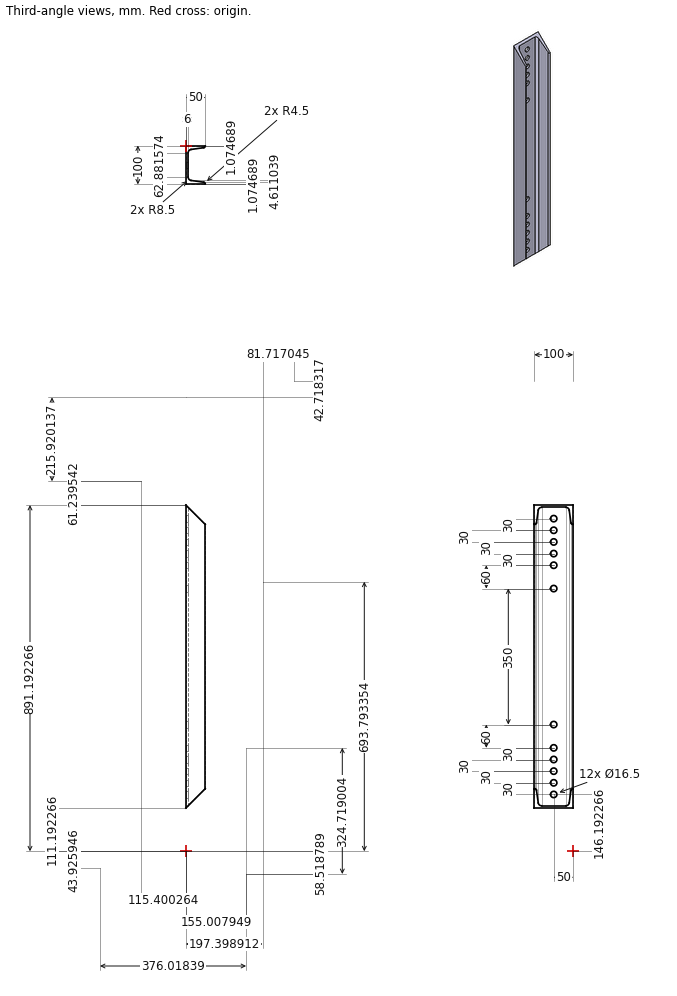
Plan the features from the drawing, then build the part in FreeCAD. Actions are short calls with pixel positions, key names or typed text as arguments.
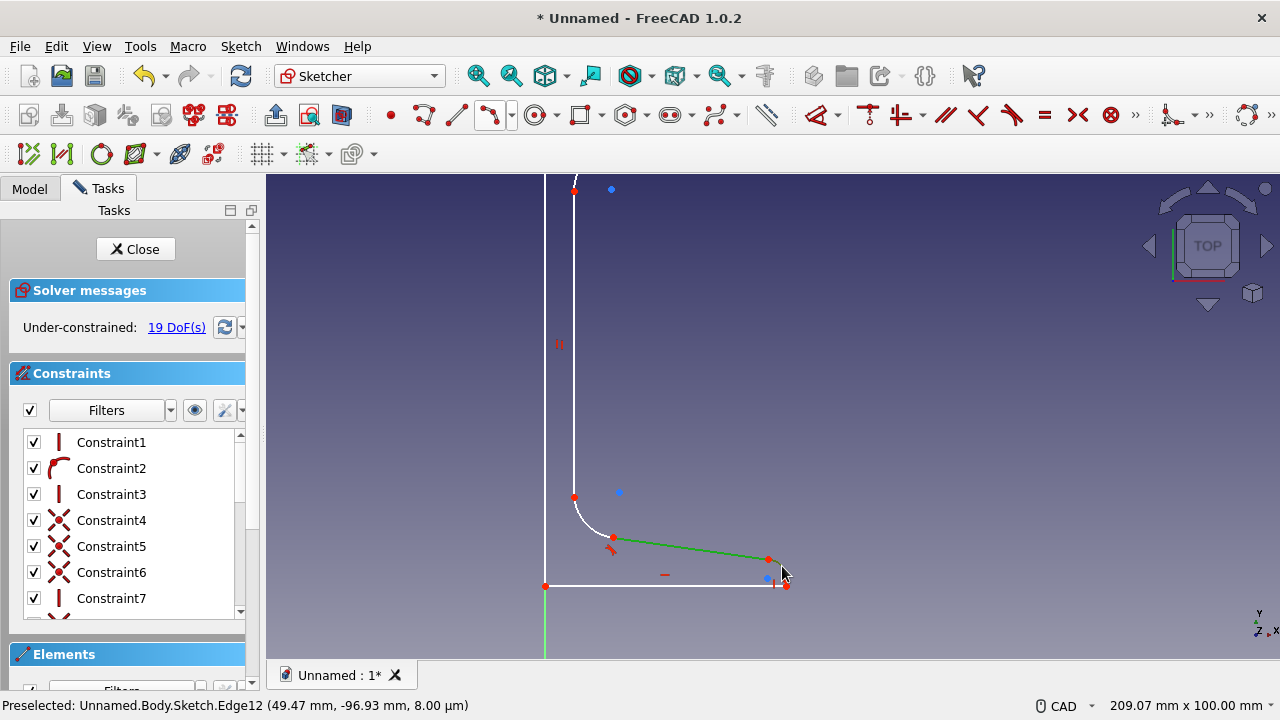
click(1012, 116)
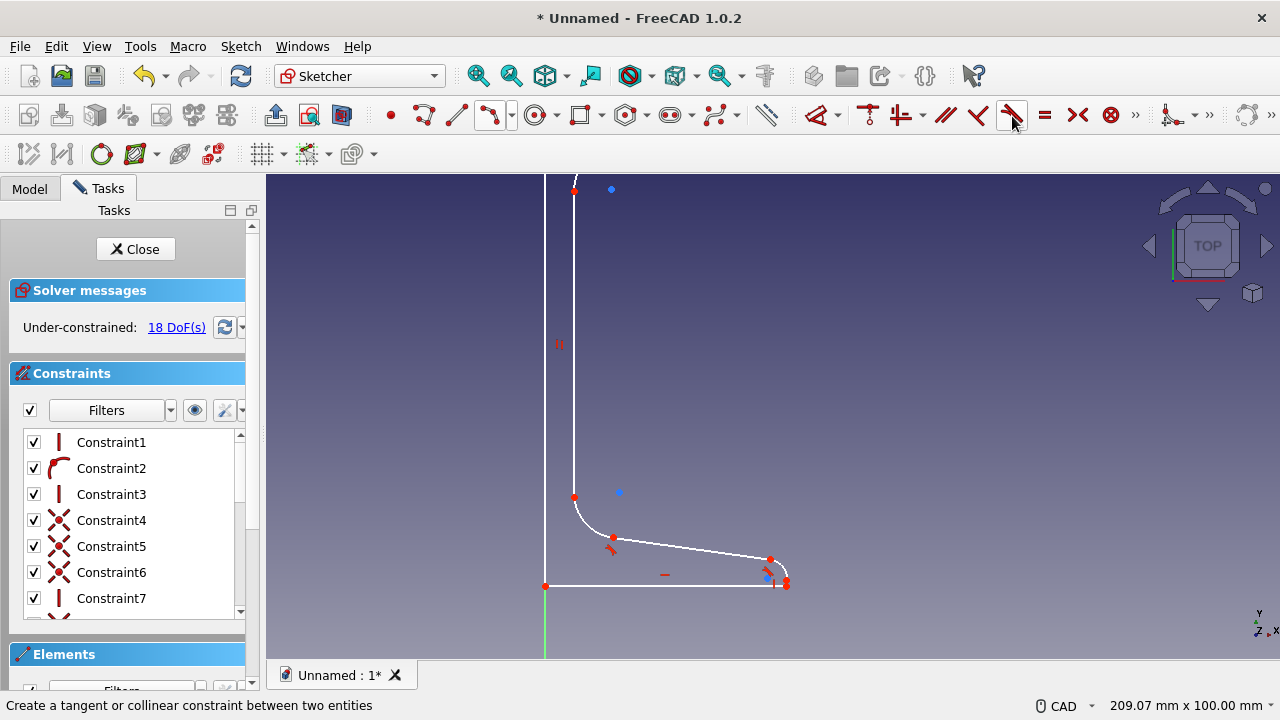
click(574, 406)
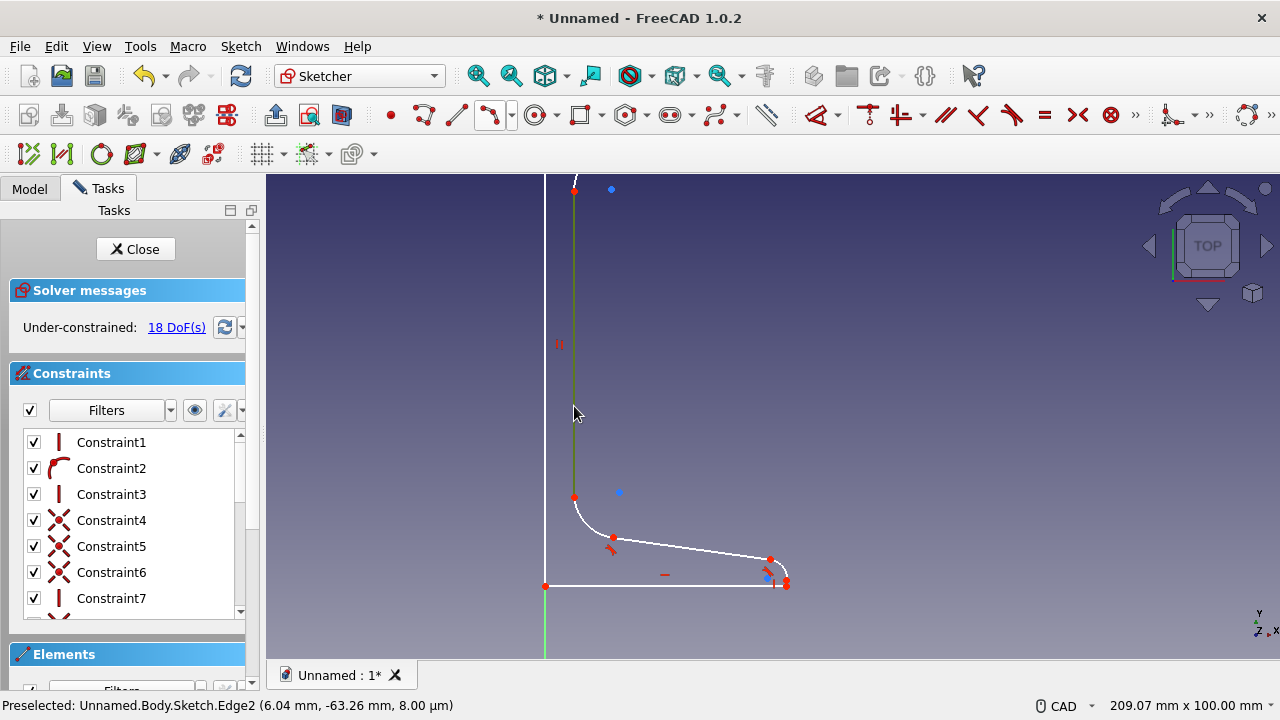
click(580, 515)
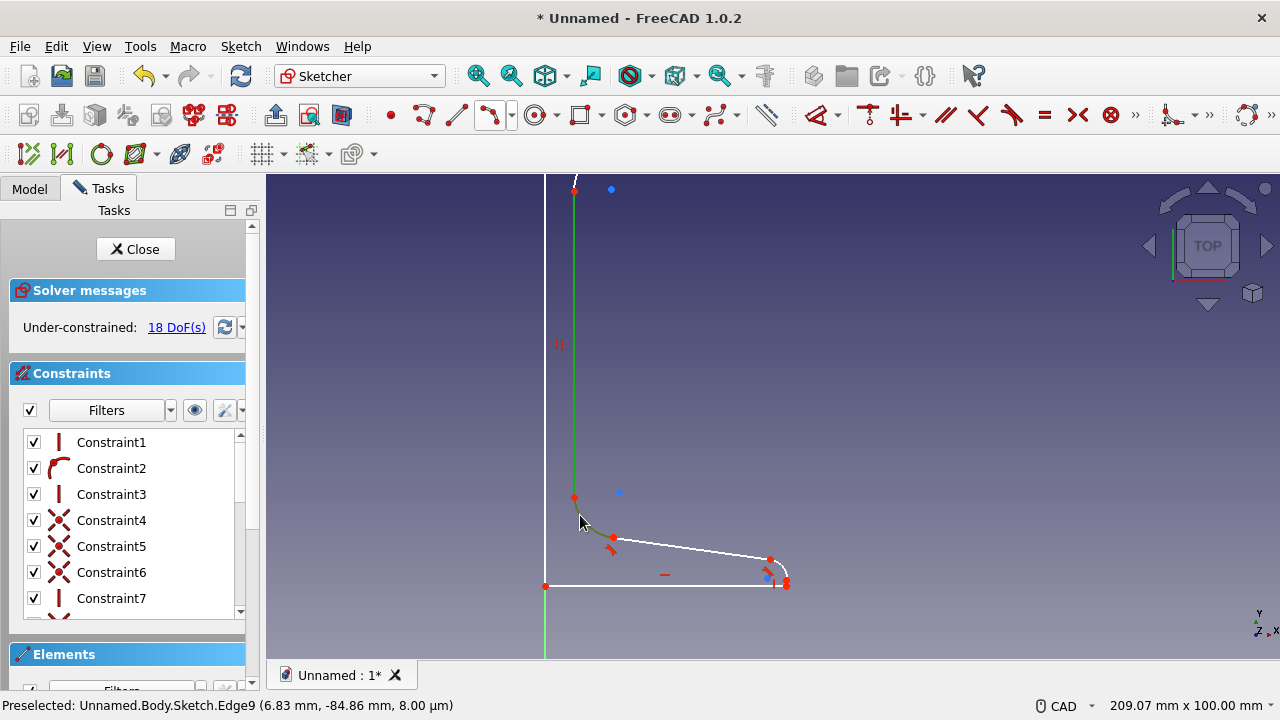
click(1012, 116)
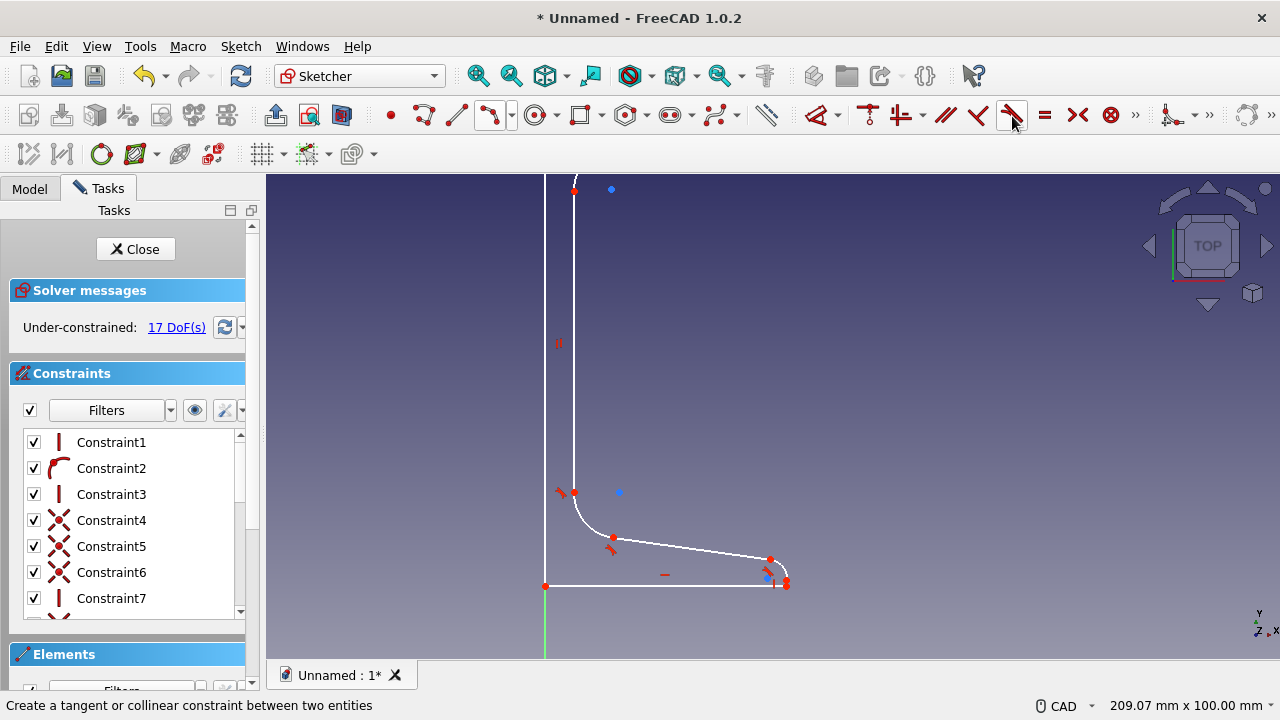
click(574, 403)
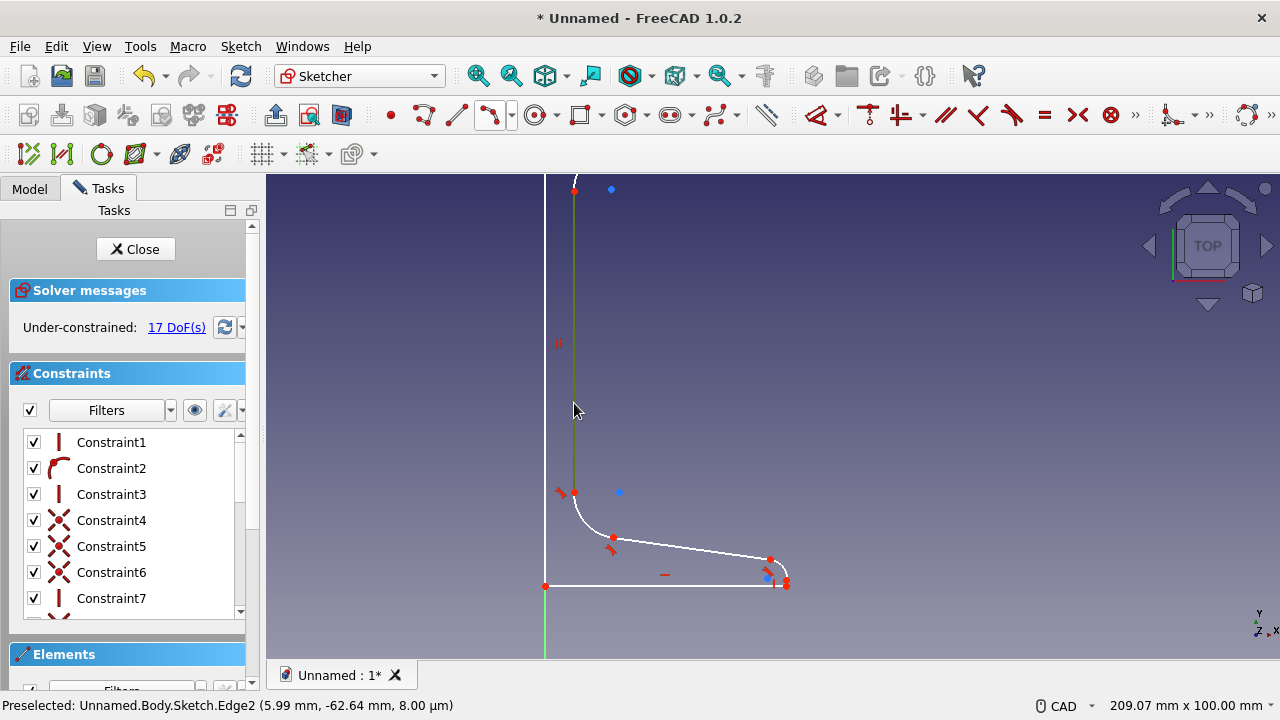
scroll(782, 567, down, 2)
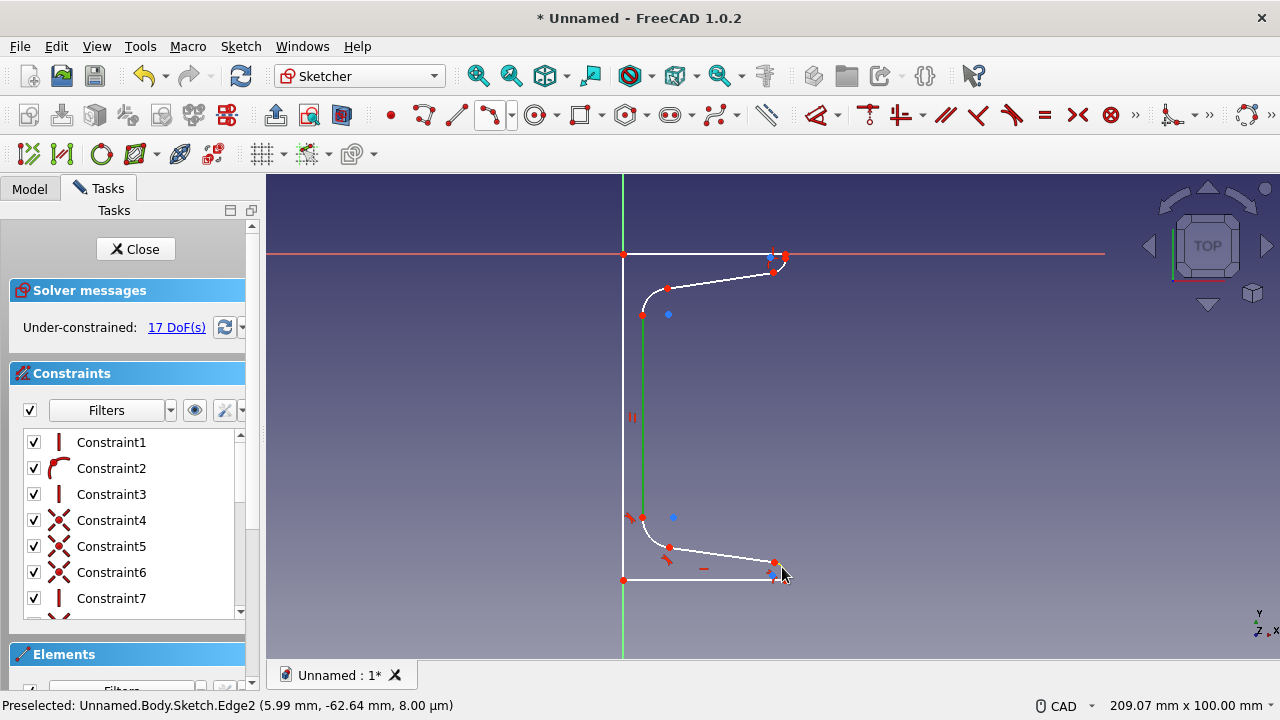
click(656, 292)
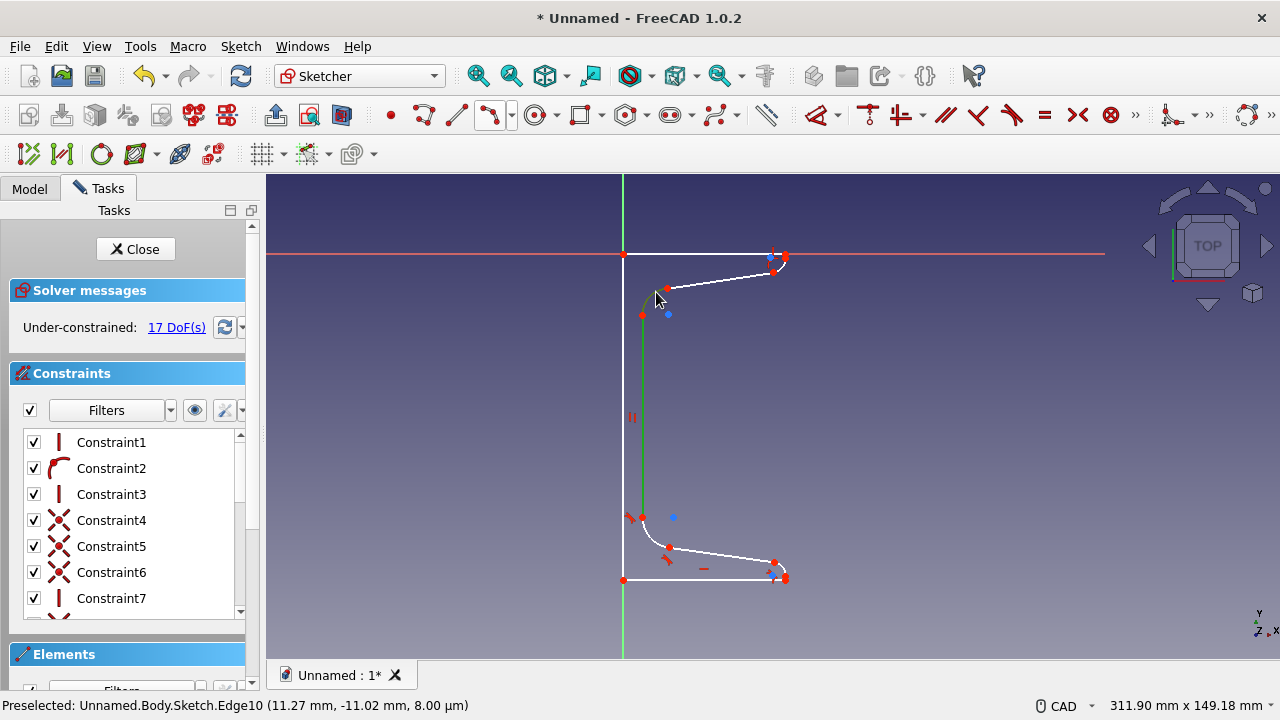
click(1012, 116)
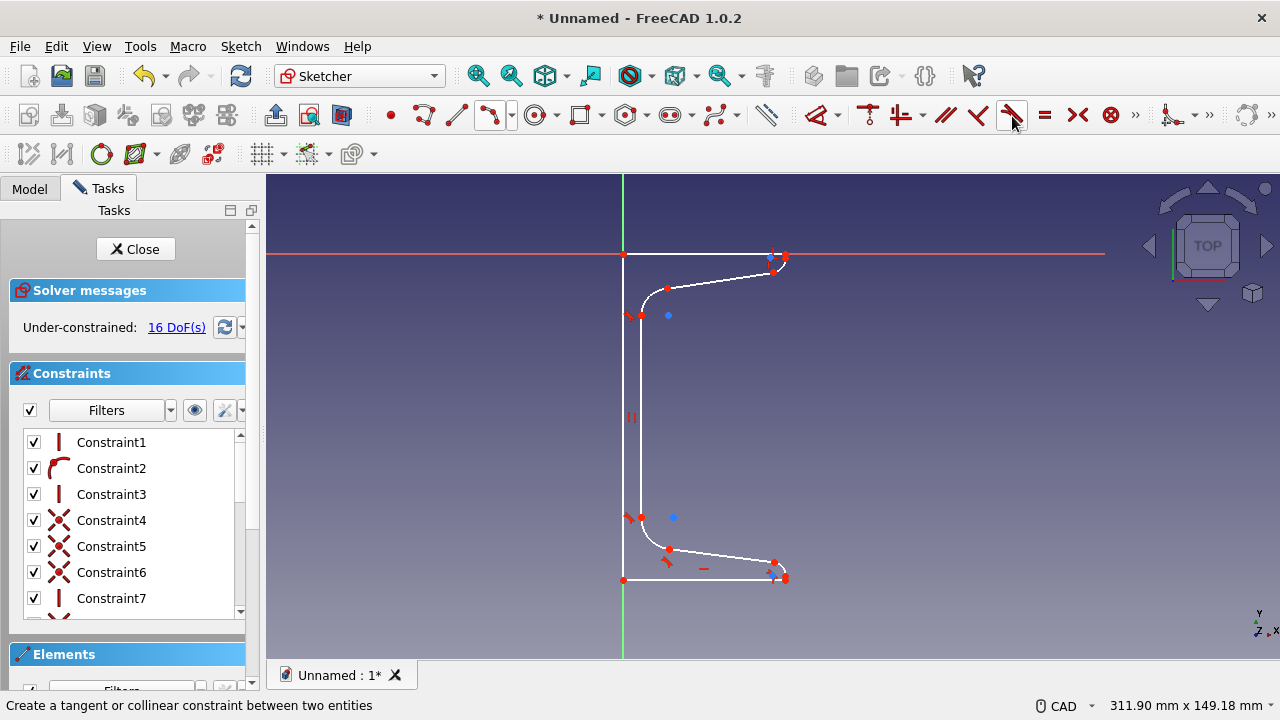
click(699, 284)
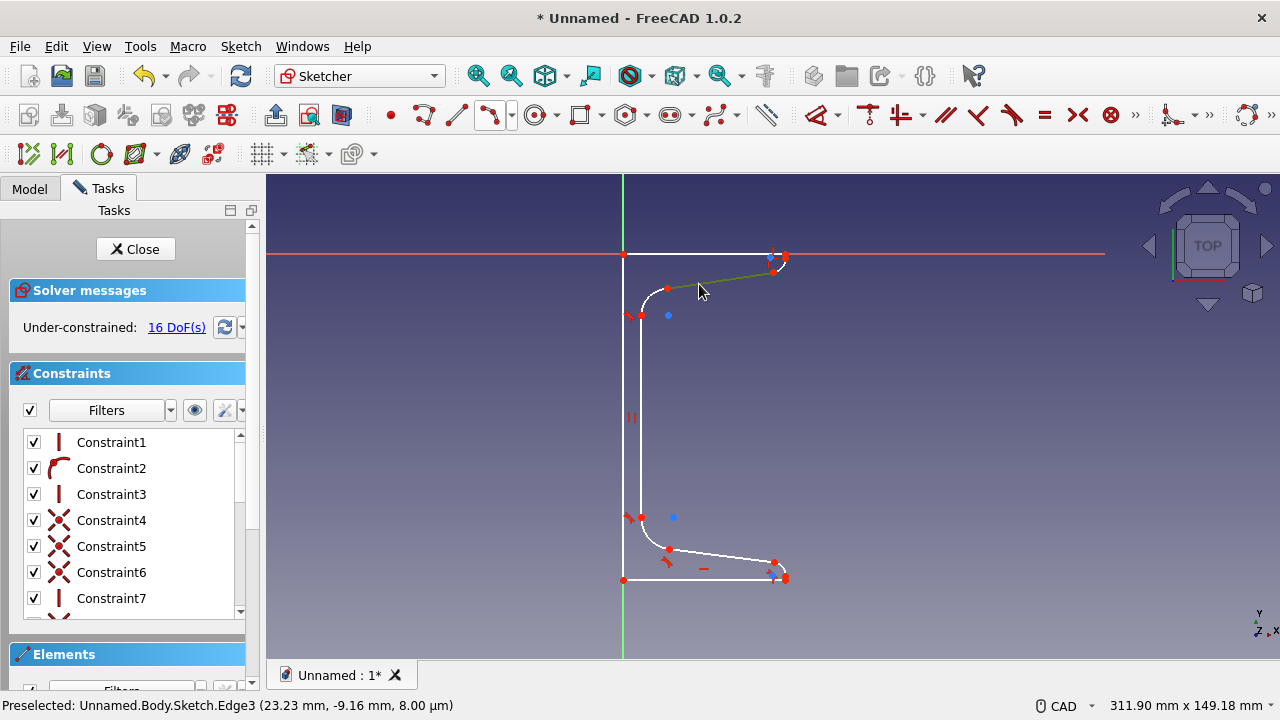
click(655, 292)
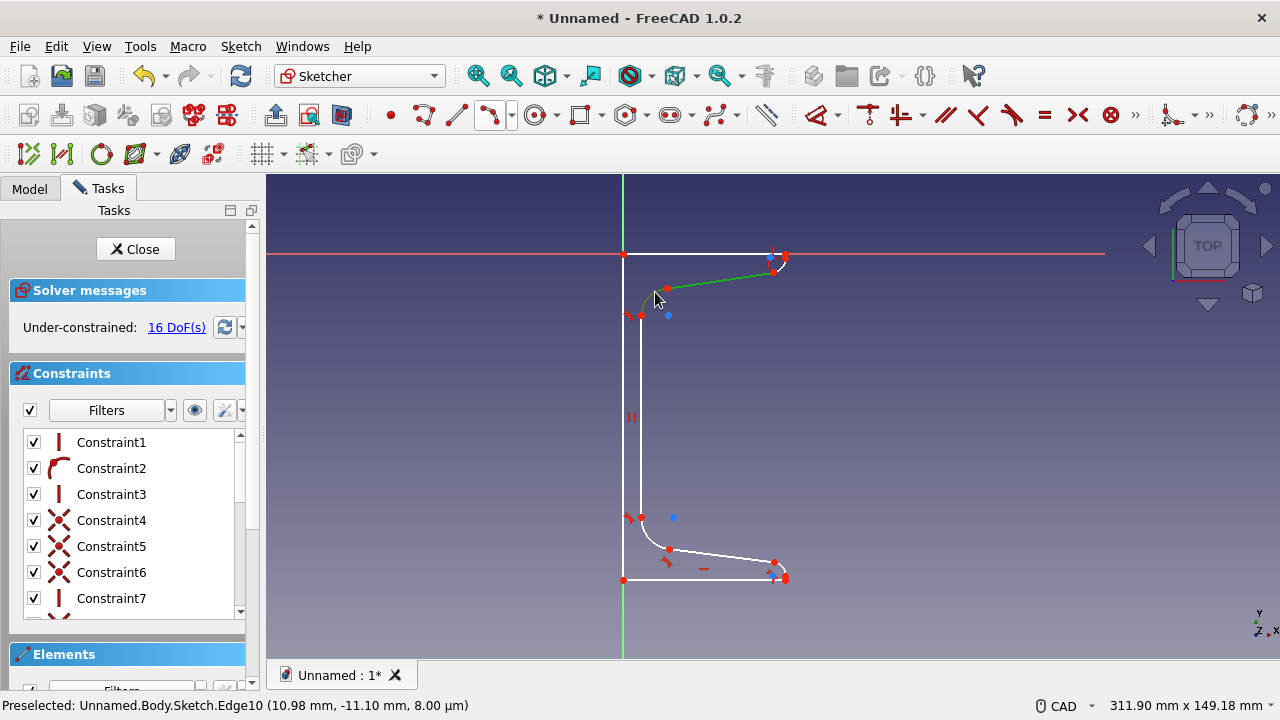
click(1012, 116)